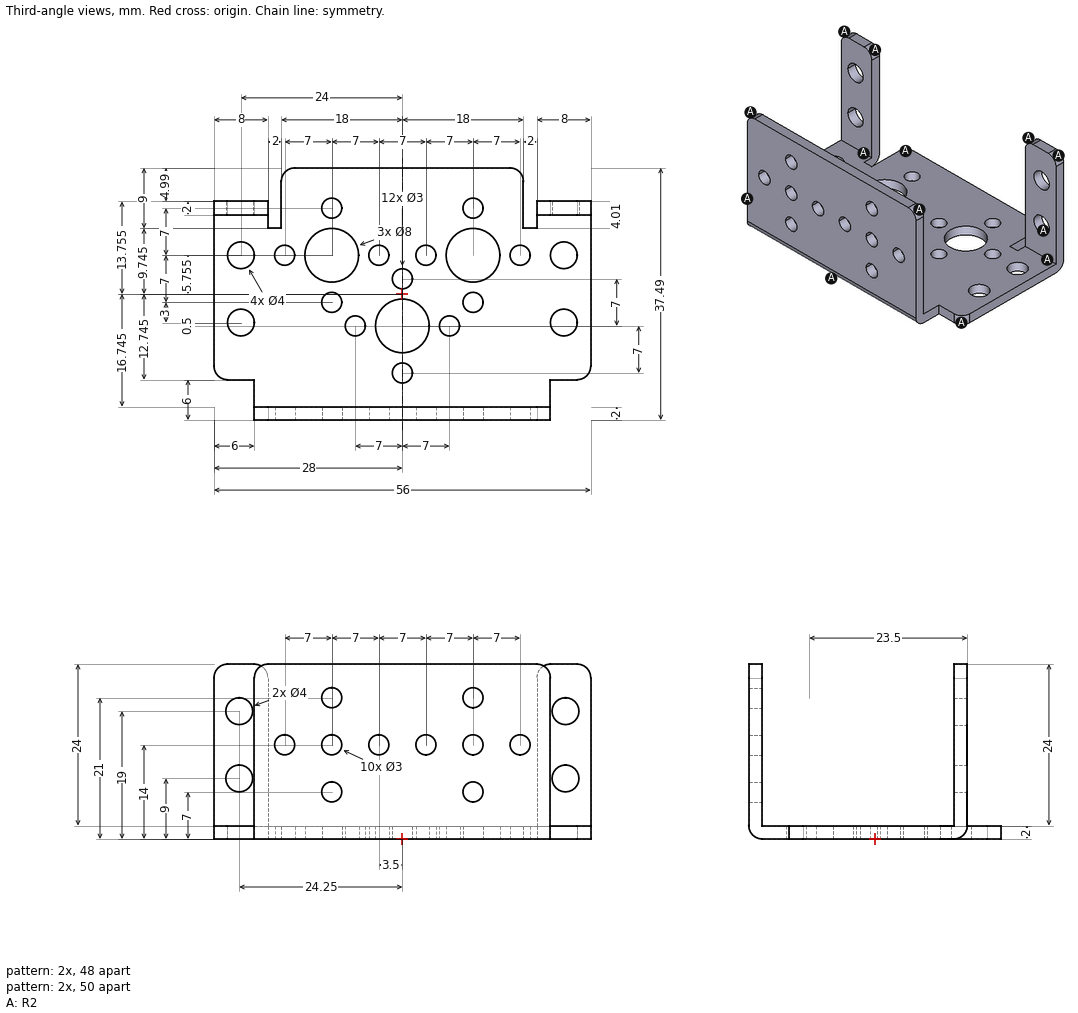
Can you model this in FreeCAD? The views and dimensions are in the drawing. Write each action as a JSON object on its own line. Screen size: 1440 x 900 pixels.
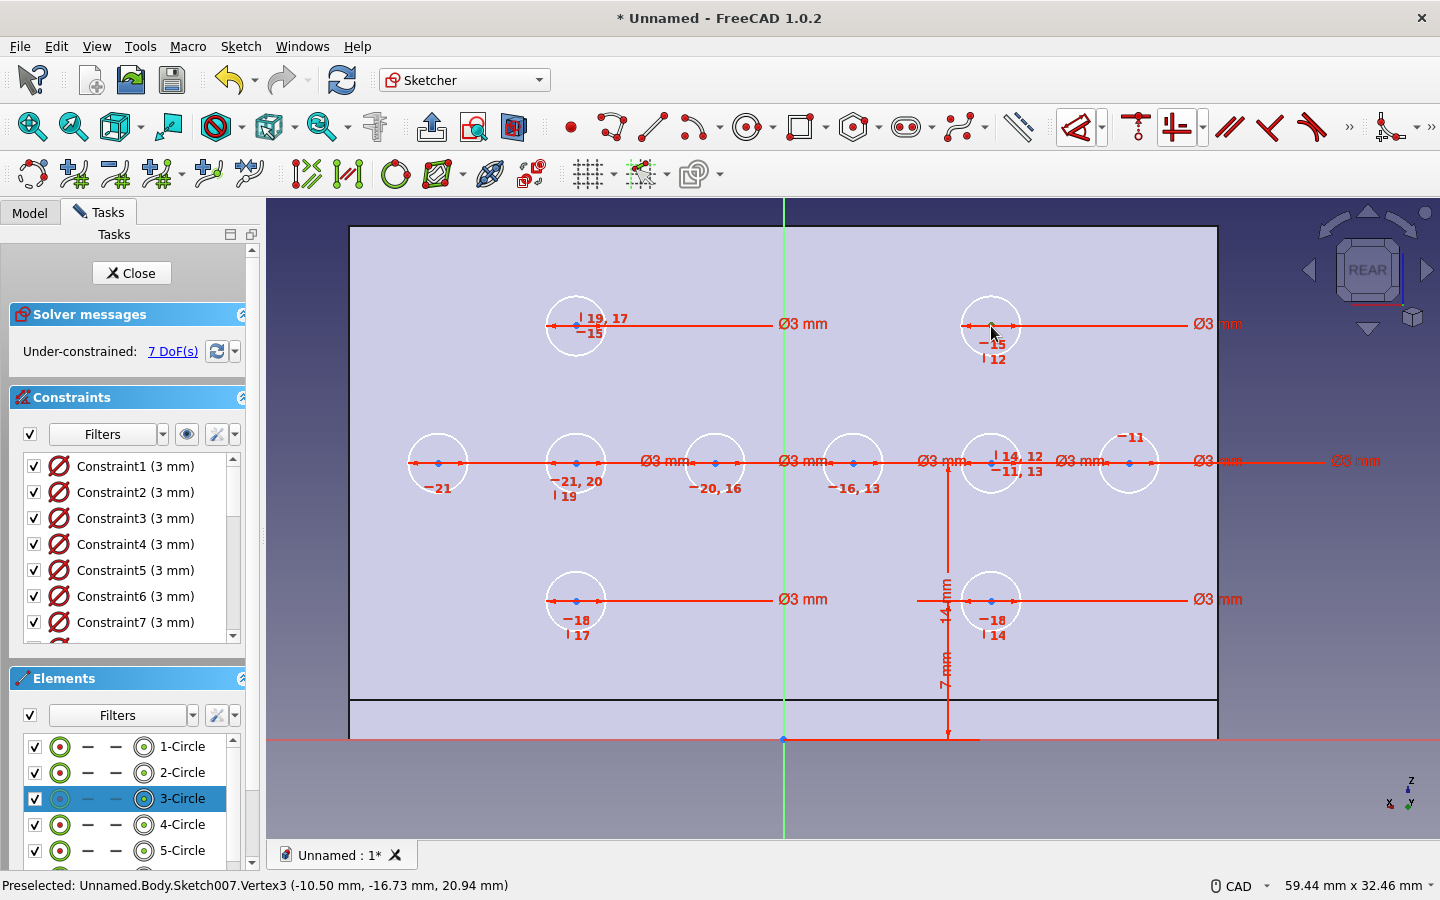
{"action": "key", "text": "i"}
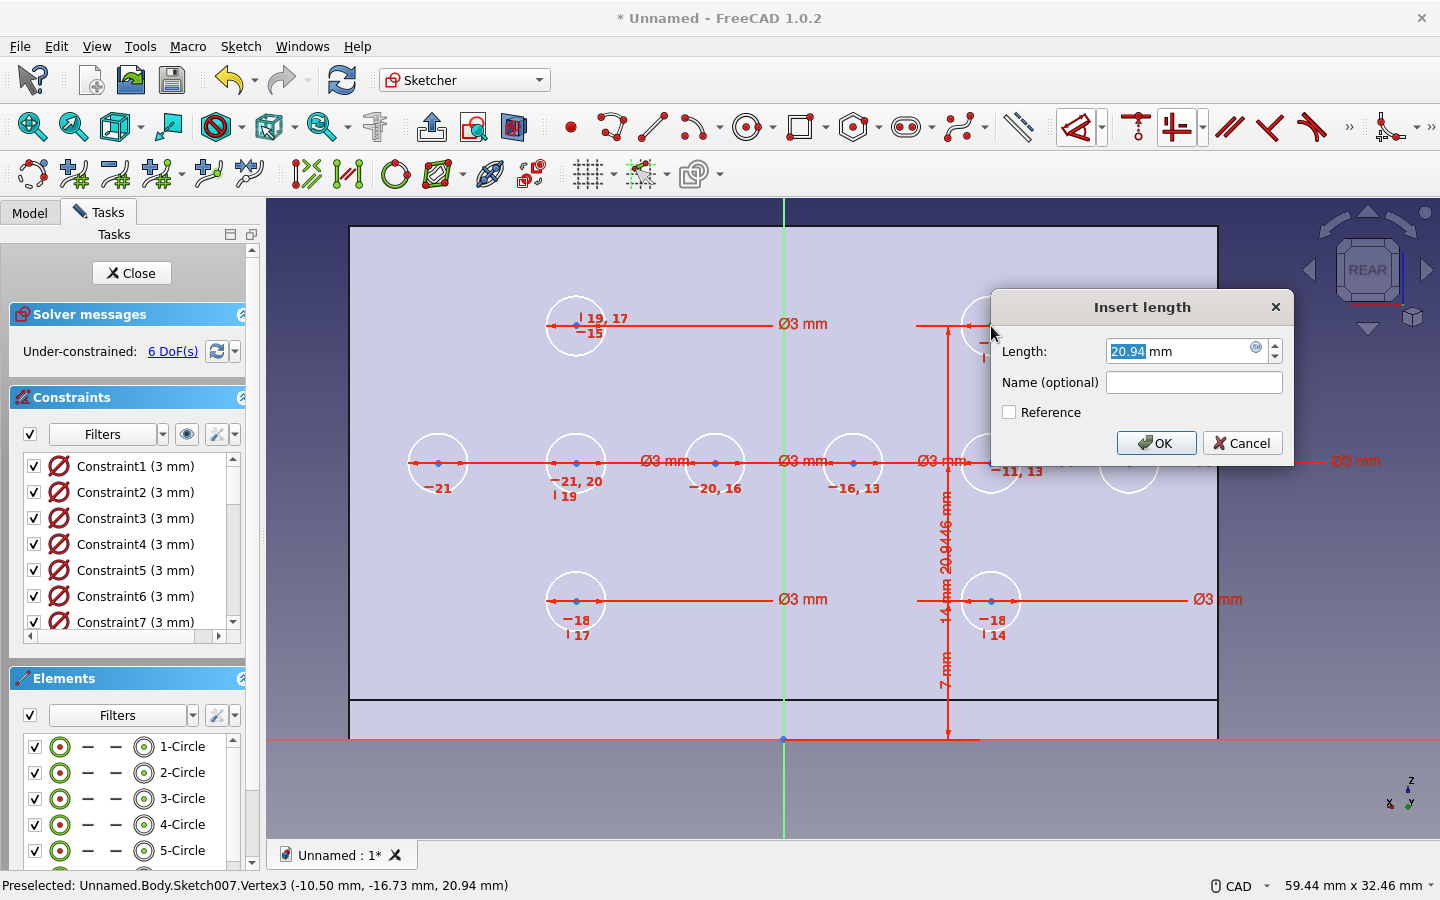
{"action": "type", "text": "21"}
{"action": "key", "text": "Return"}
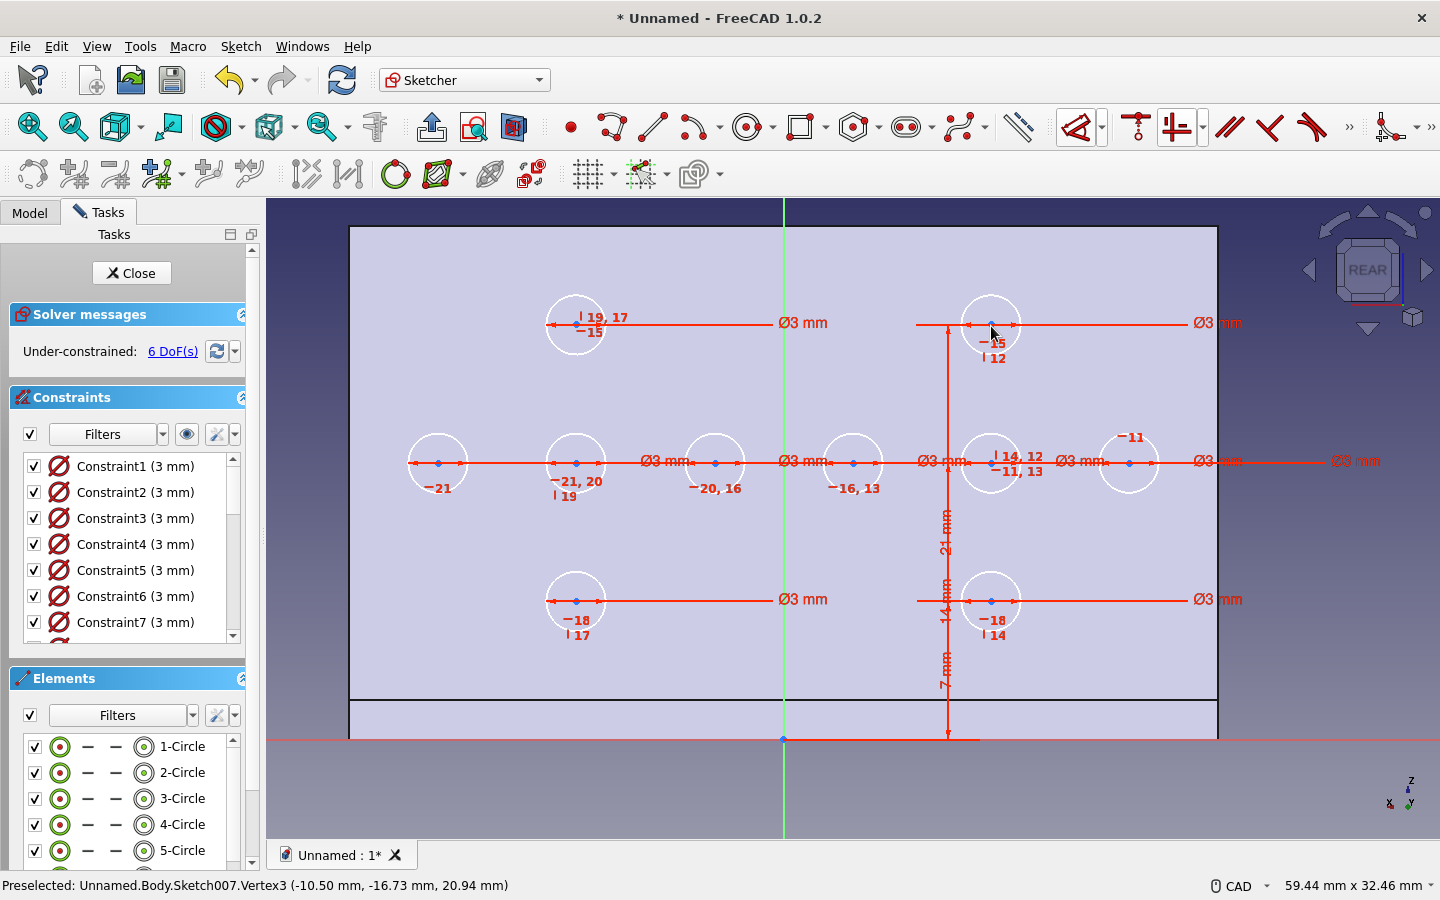
{"action": "left_click", "coordinate": [991, 463]}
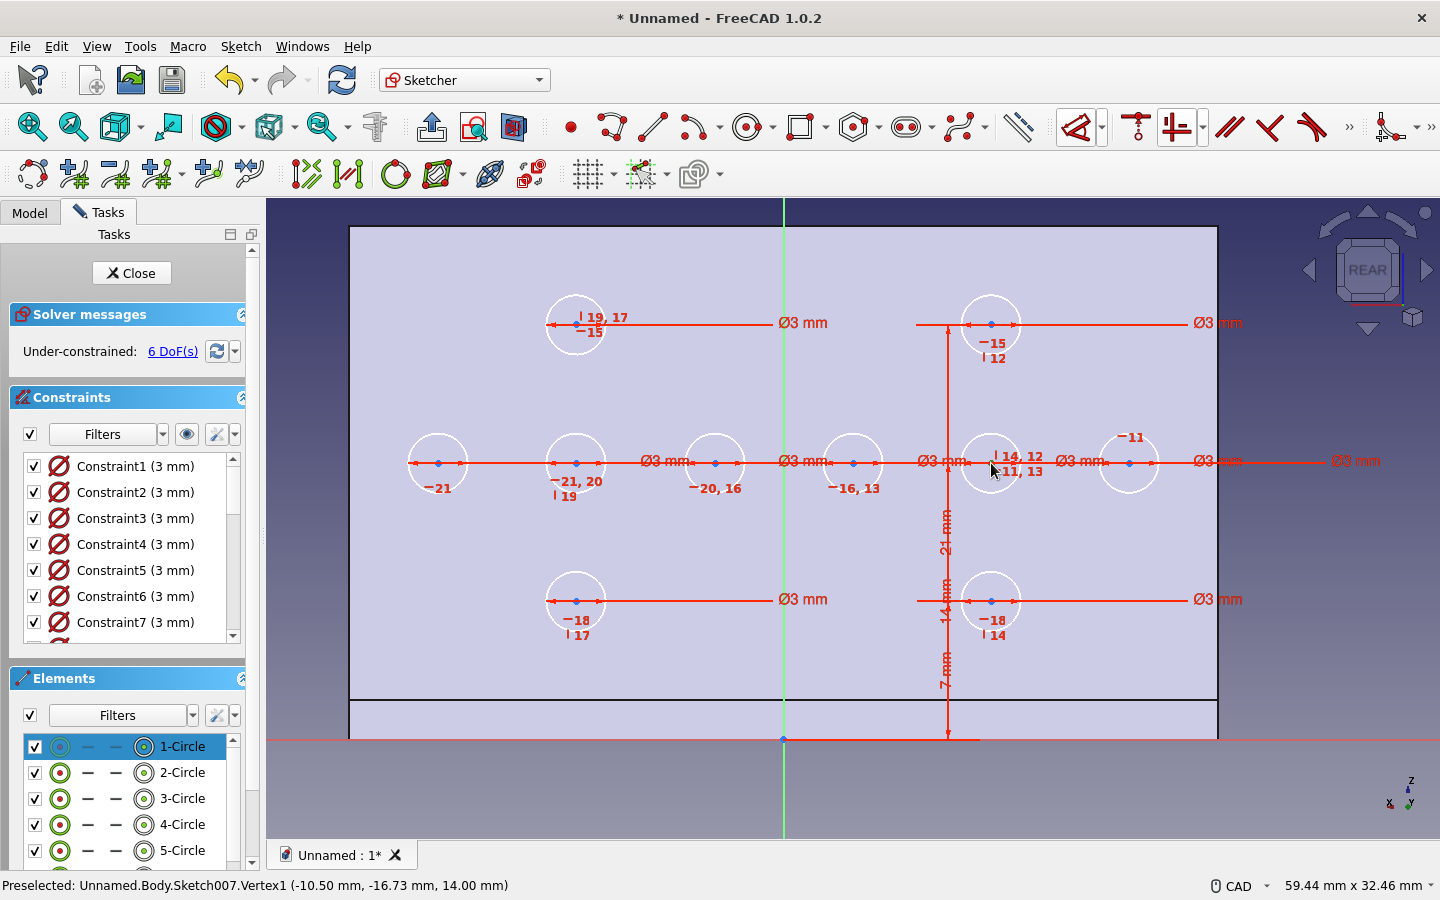
{"action": "left_click", "coordinate": [1129, 463]}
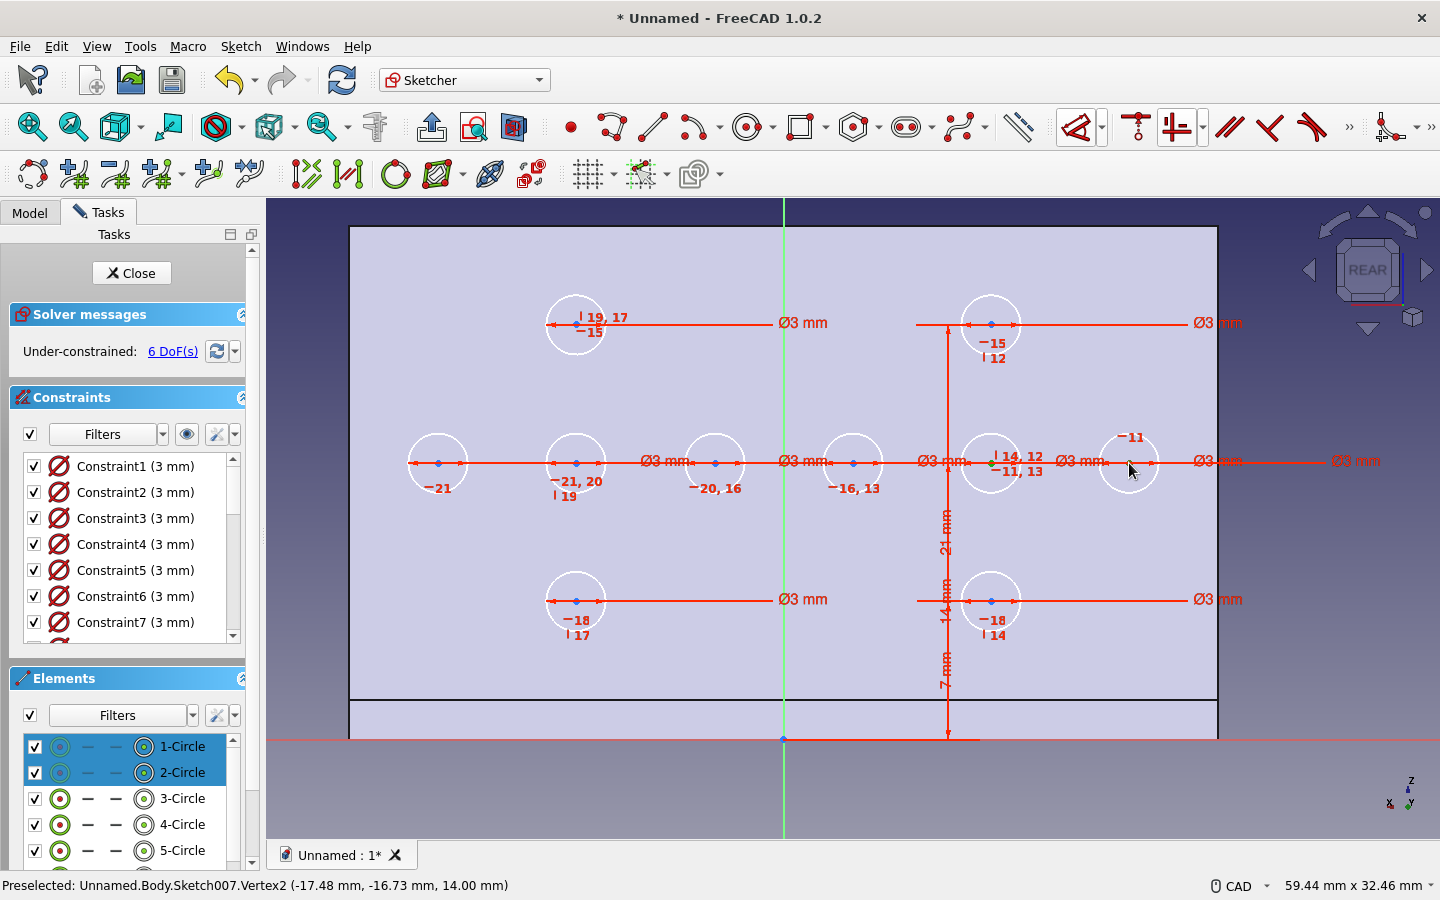
{"action": "key", "text": "l"}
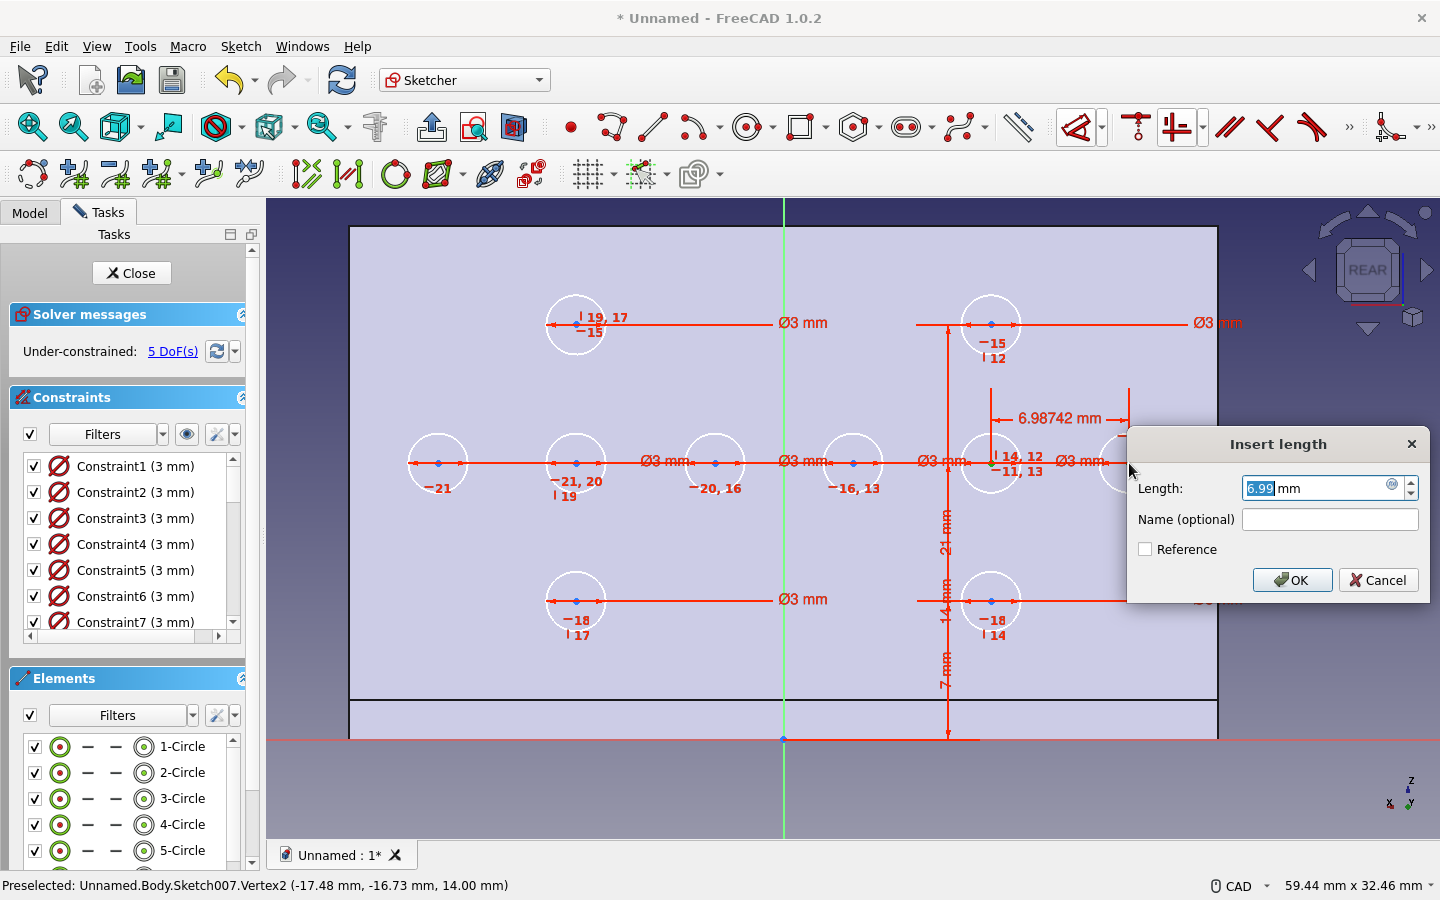
{"action": "type", "text": "7"}
{"action": "key", "text": "Return"}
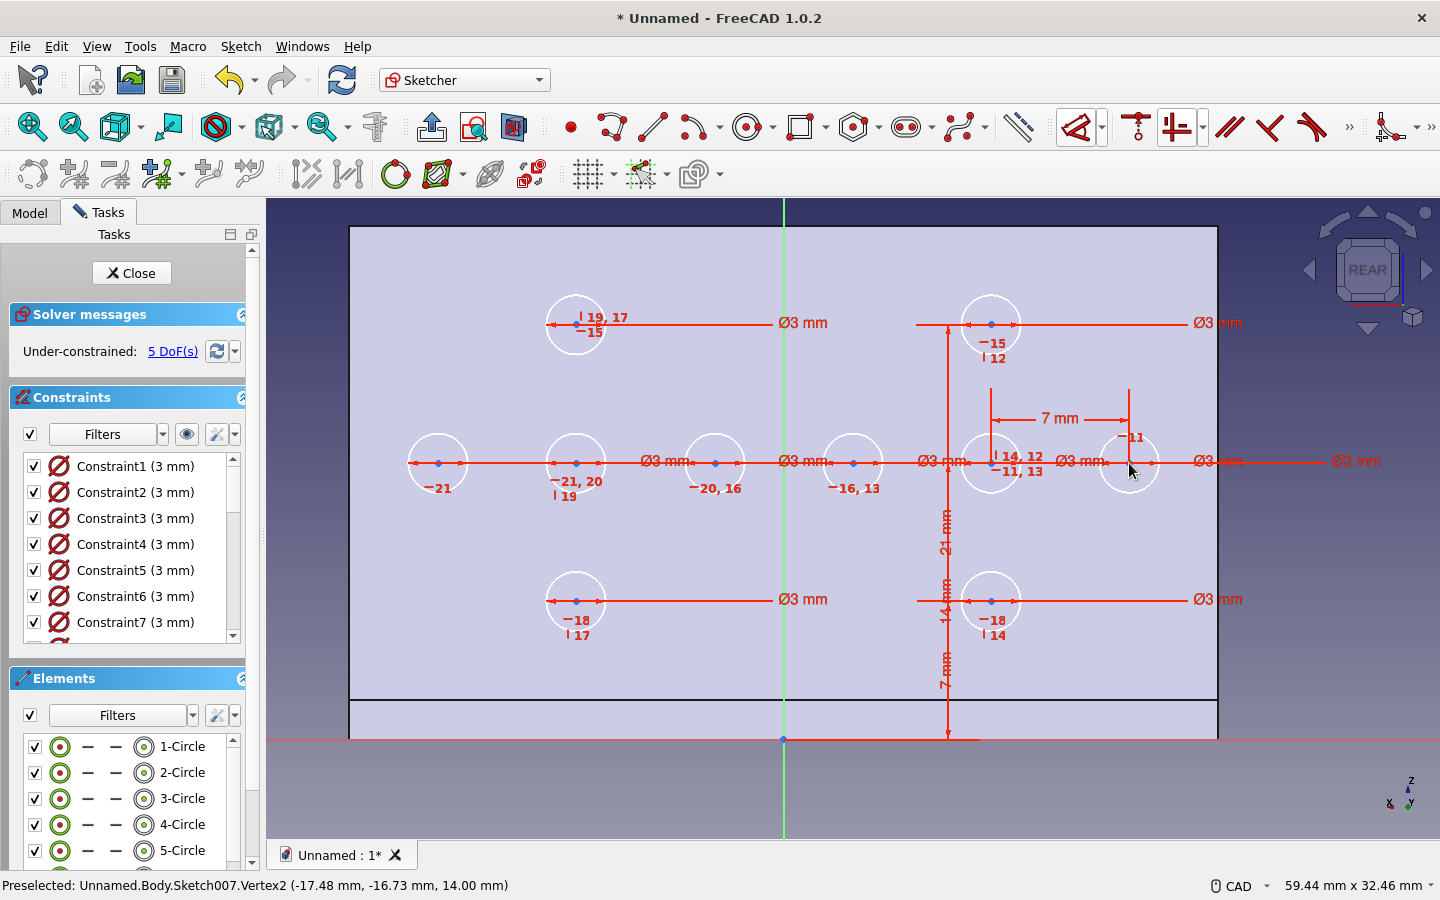
{"action": "left_click", "coordinate": [991, 463]}